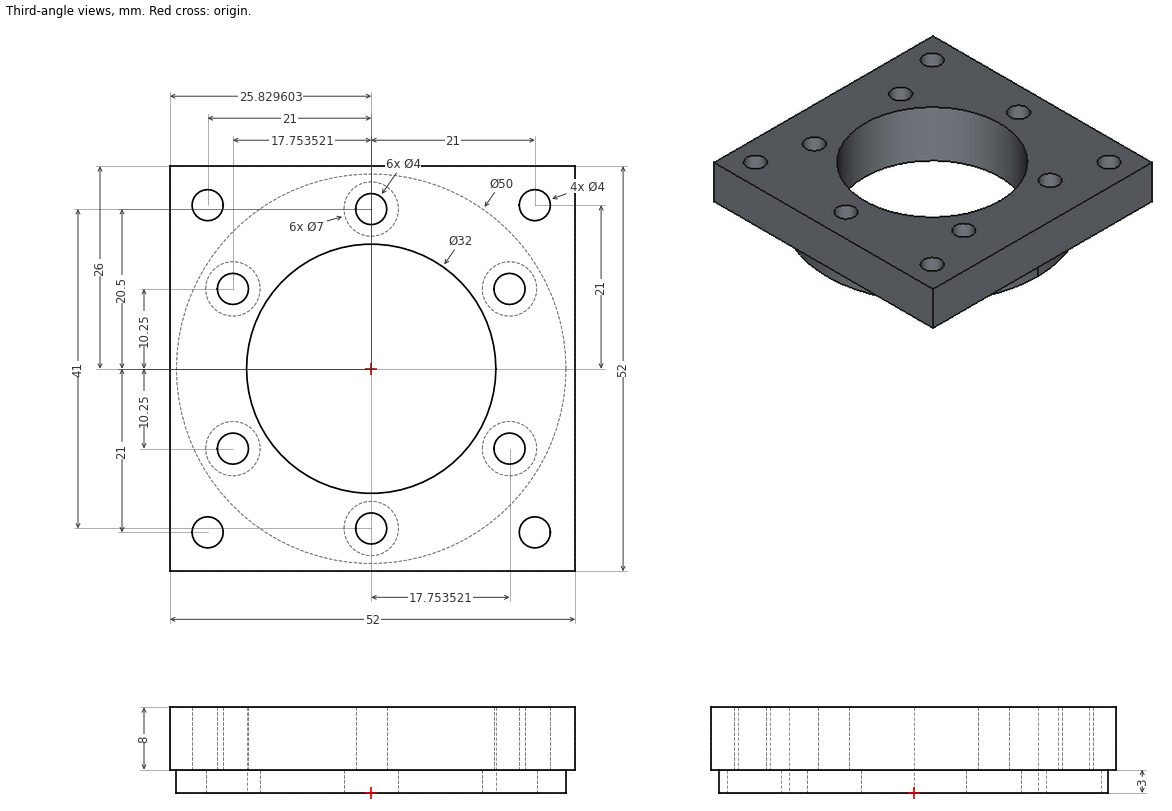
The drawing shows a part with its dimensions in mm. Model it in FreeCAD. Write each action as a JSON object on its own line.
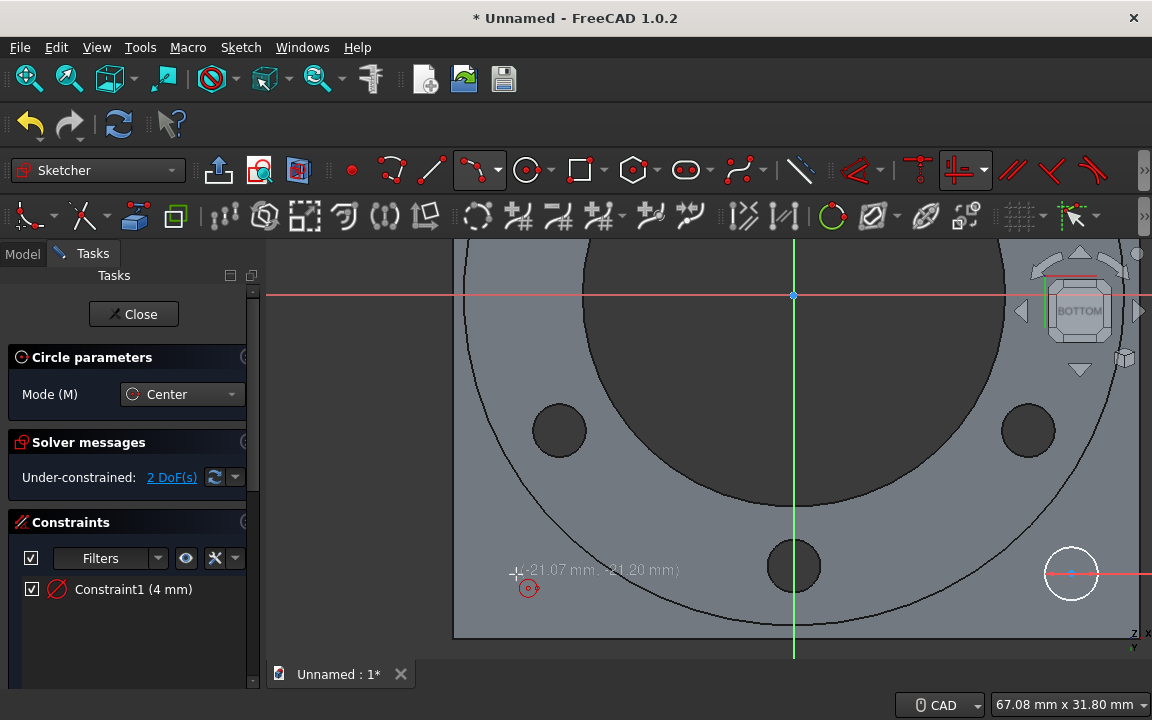
{"action": "left_click", "coordinate": [517, 573]}
{"action": "mouse_move", "coordinate": [535, 554]}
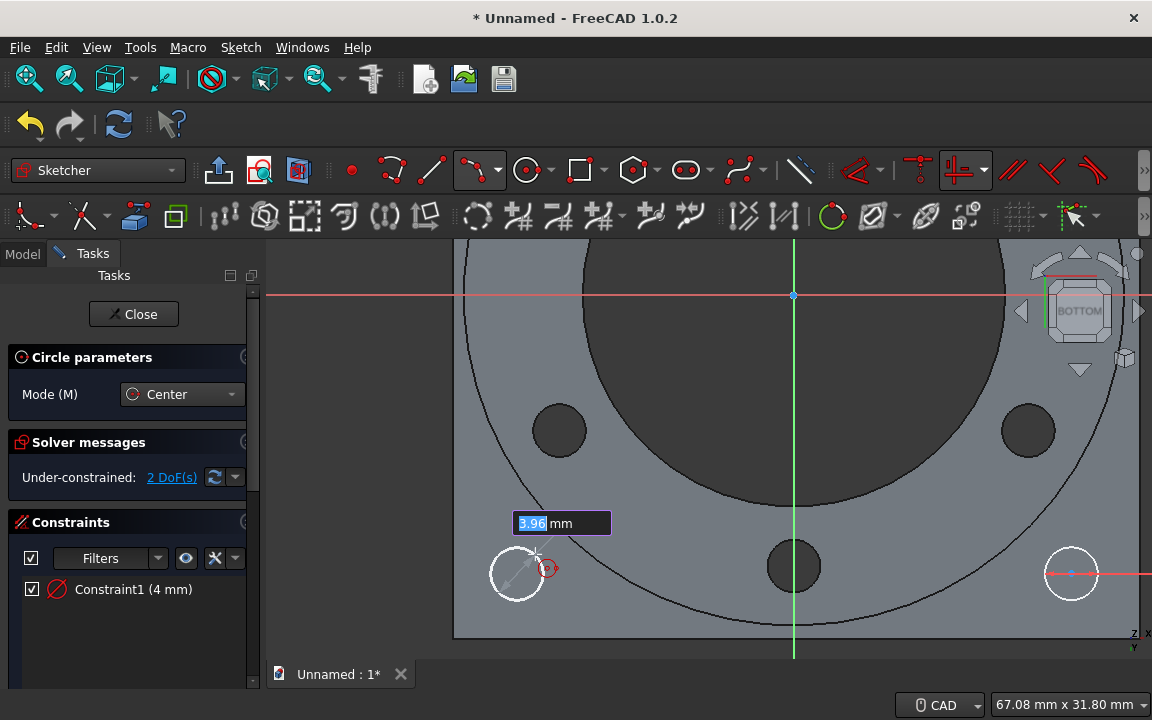
{"action": "type", "text": "4"}
{"action": "key", "text": "Return"}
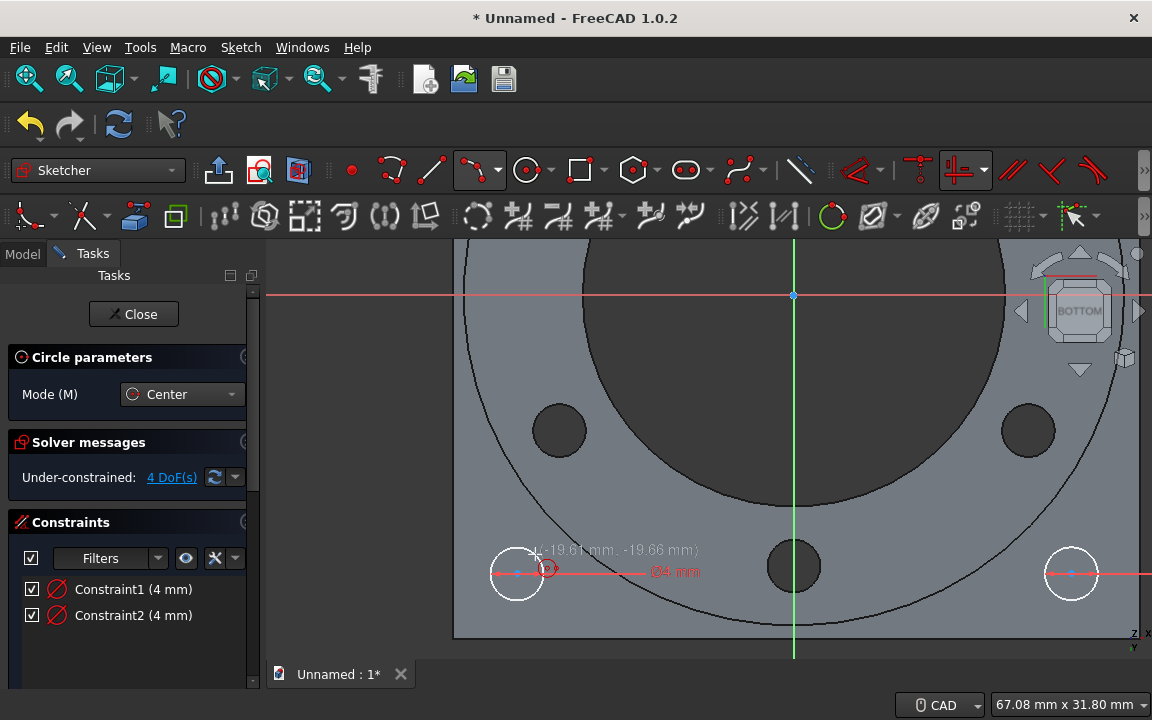
{"action": "scroll", "coordinate": [515, 574], "scroll_direction": "down", "scroll_amount": 4}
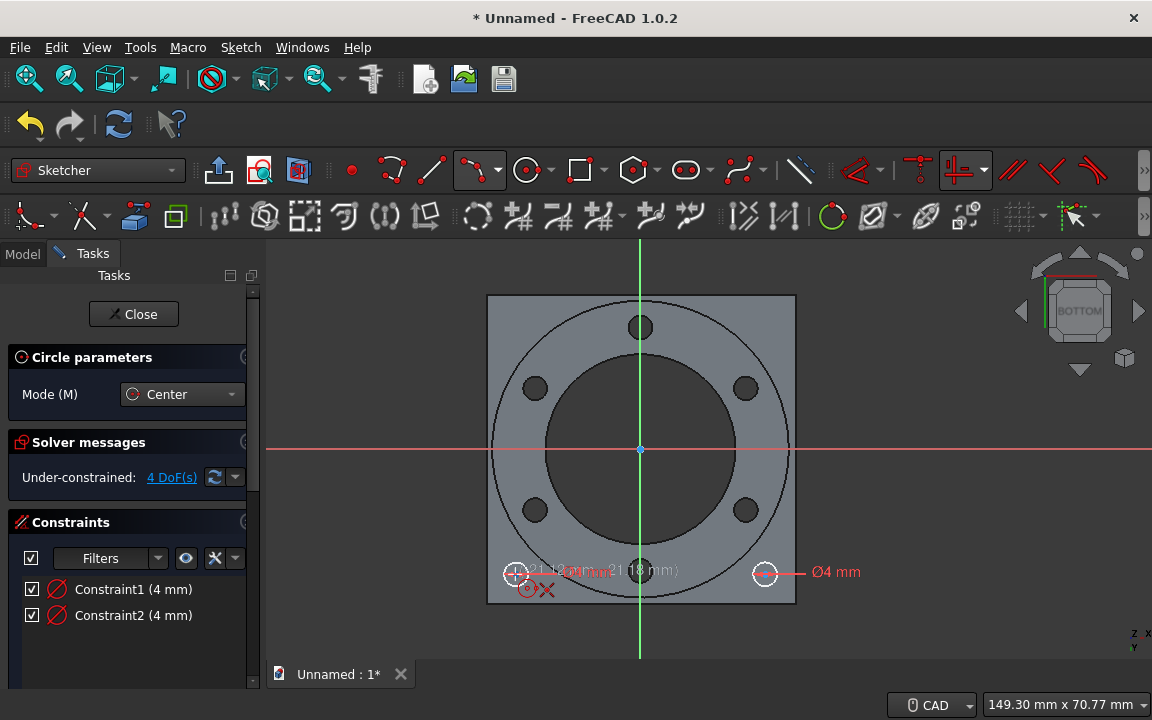
{"action": "scroll", "coordinate": [516, 325], "scroll_direction": "up", "scroll_amount": 4}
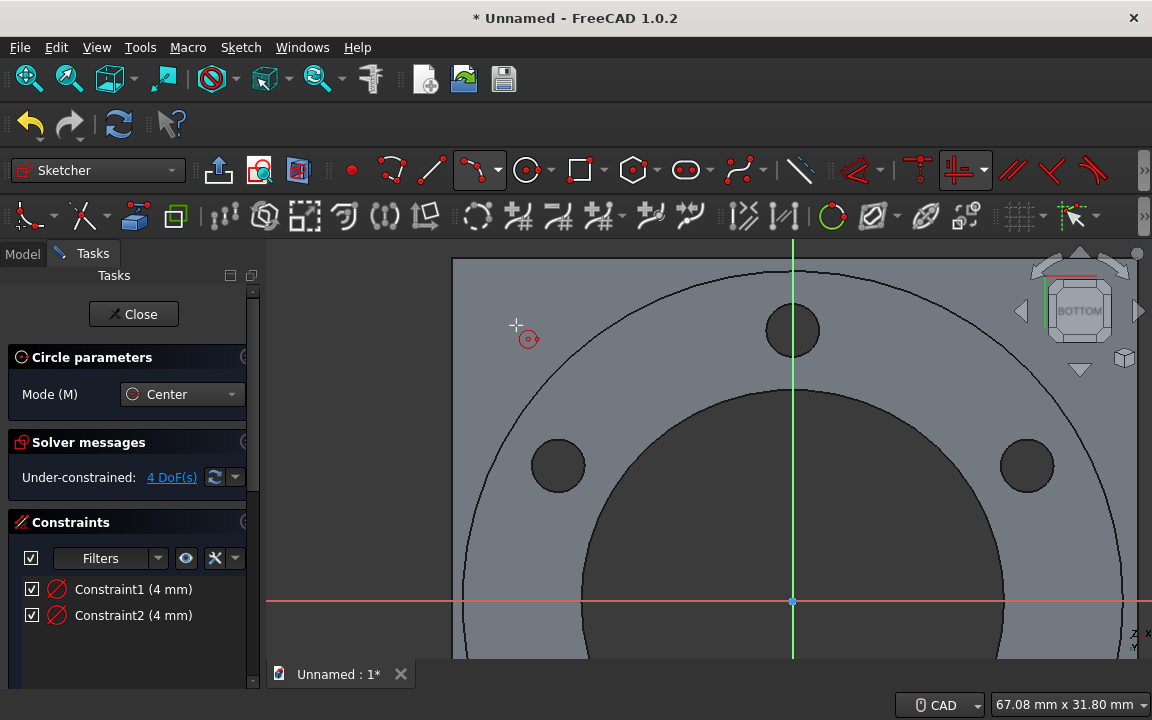
{"action": "left_click", "coordinate": [515, 324]}
{"action": "mouse_move", "coordinate": [534, 305]}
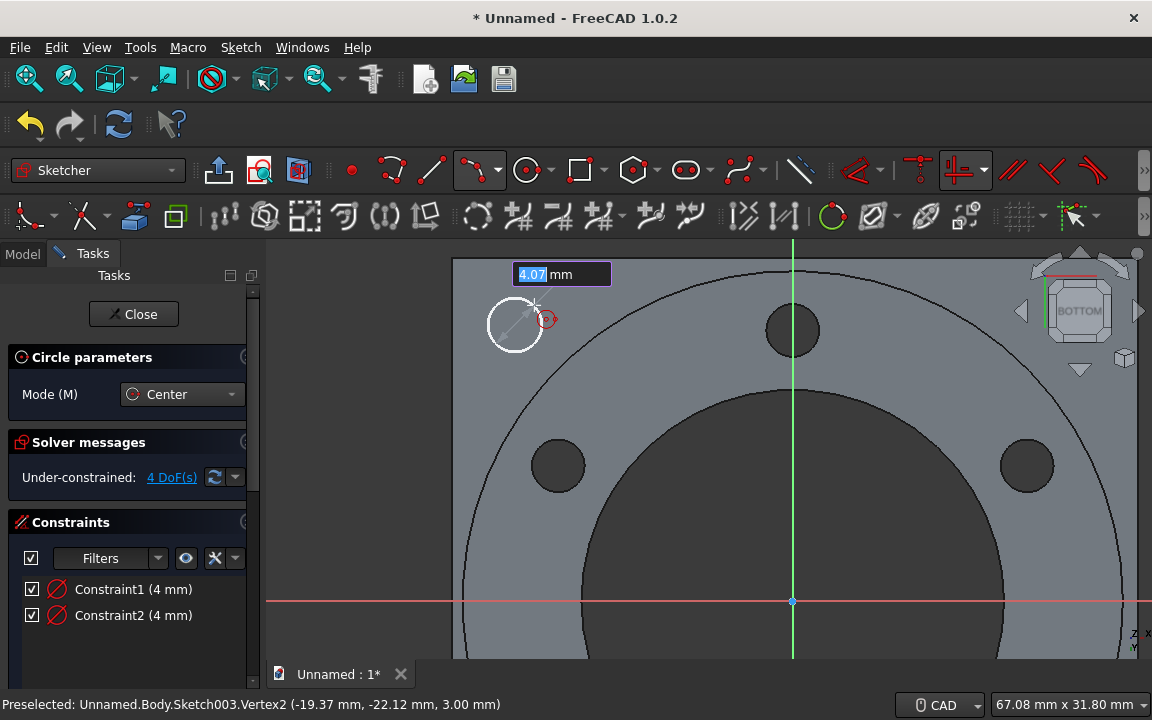
{"action": "type", "text": "4"}
{"action": "key", "text": "Return"}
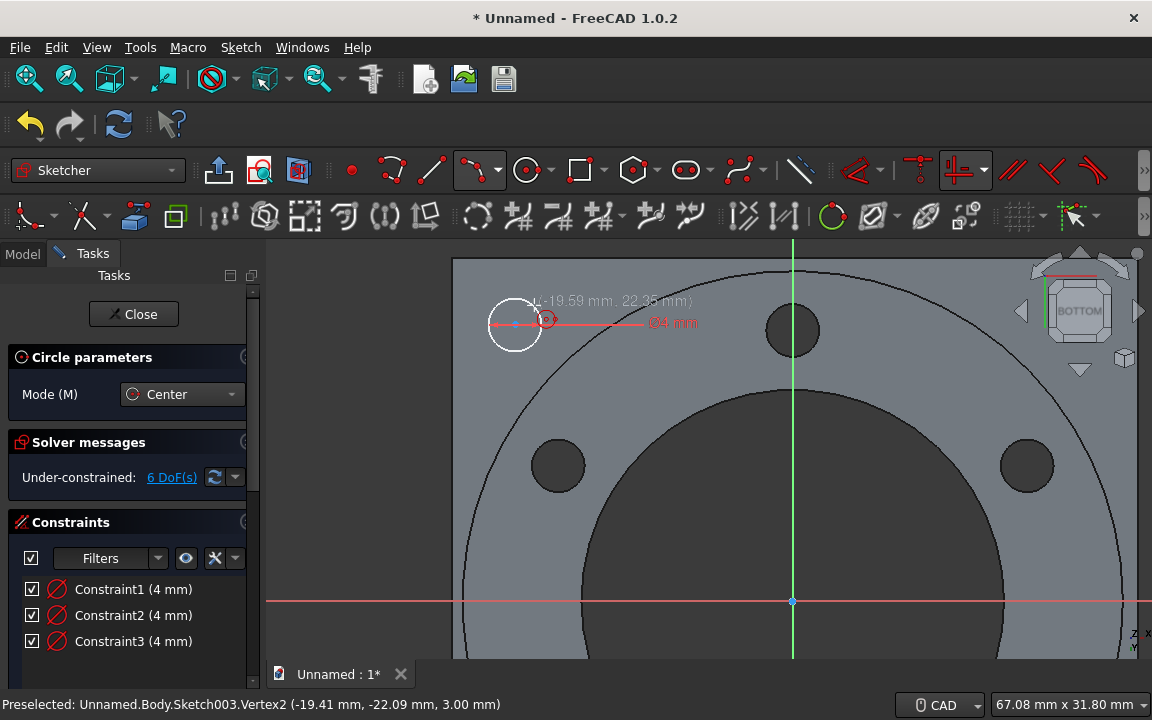
{"action": "scroll", "coordinate": [516, 325], "scroll_direction": "down", "scroll_amount": 4}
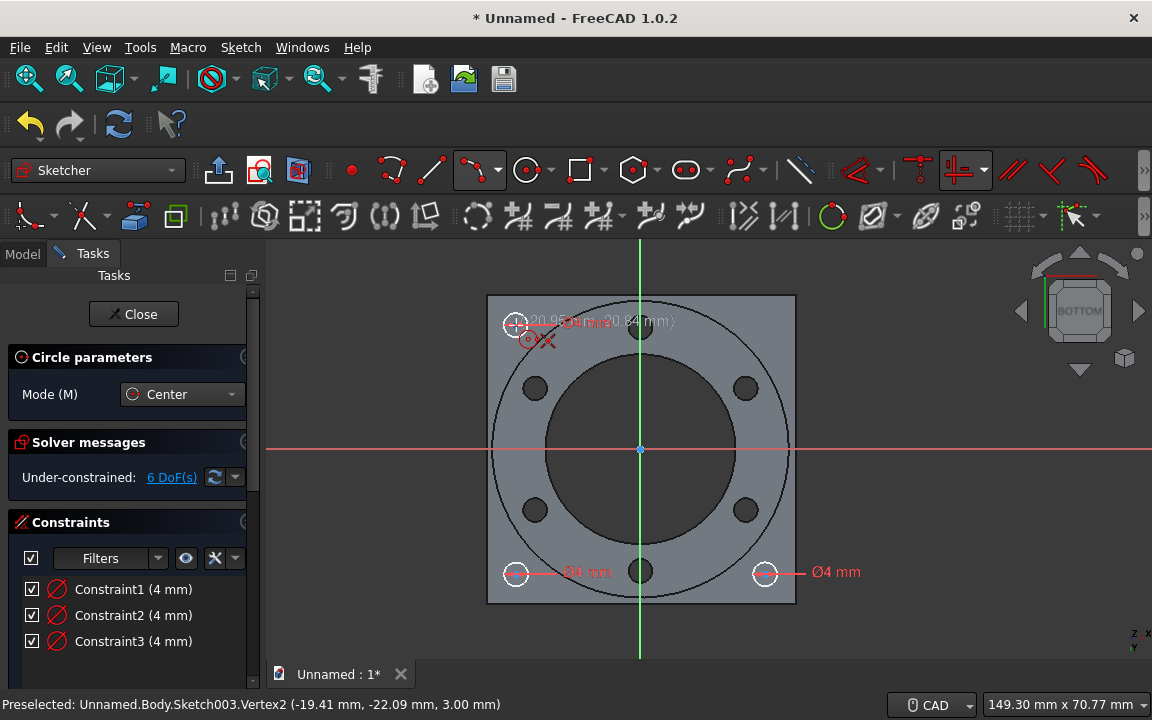
{"action": "scroll", "coordinate": [765, 325], "scroll_direction": "up", "scroll_amount": 4}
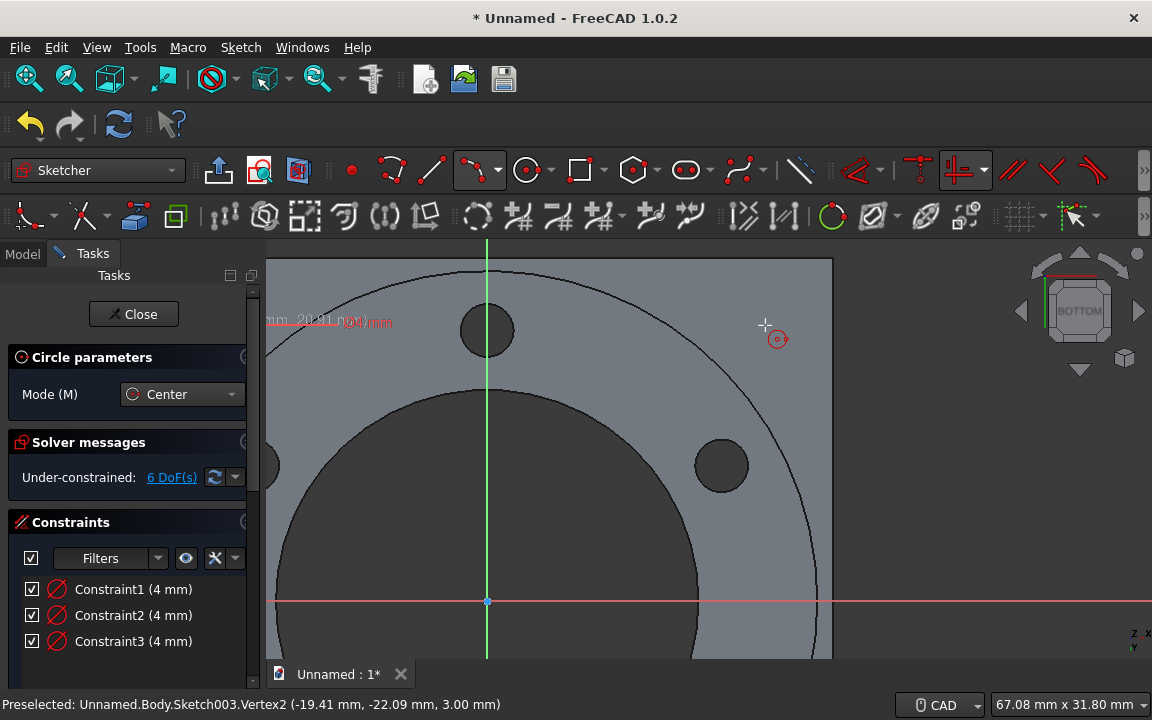
{"action": "left_click", "coordinate": [765, 324]}
{"action": "mouse_move", "coordinate": [783, 305]}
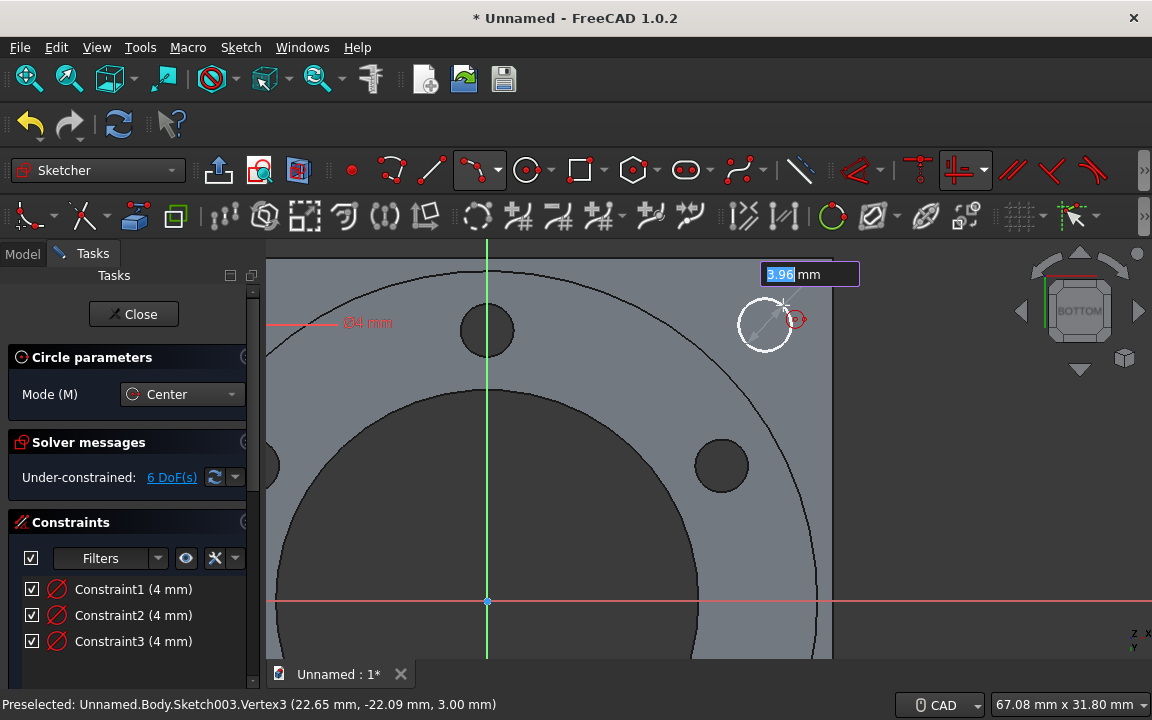
{"action": "type", "text": "4"}
{"action": "key", "text": "Return"}
{"action": "key", "text": "Escape"}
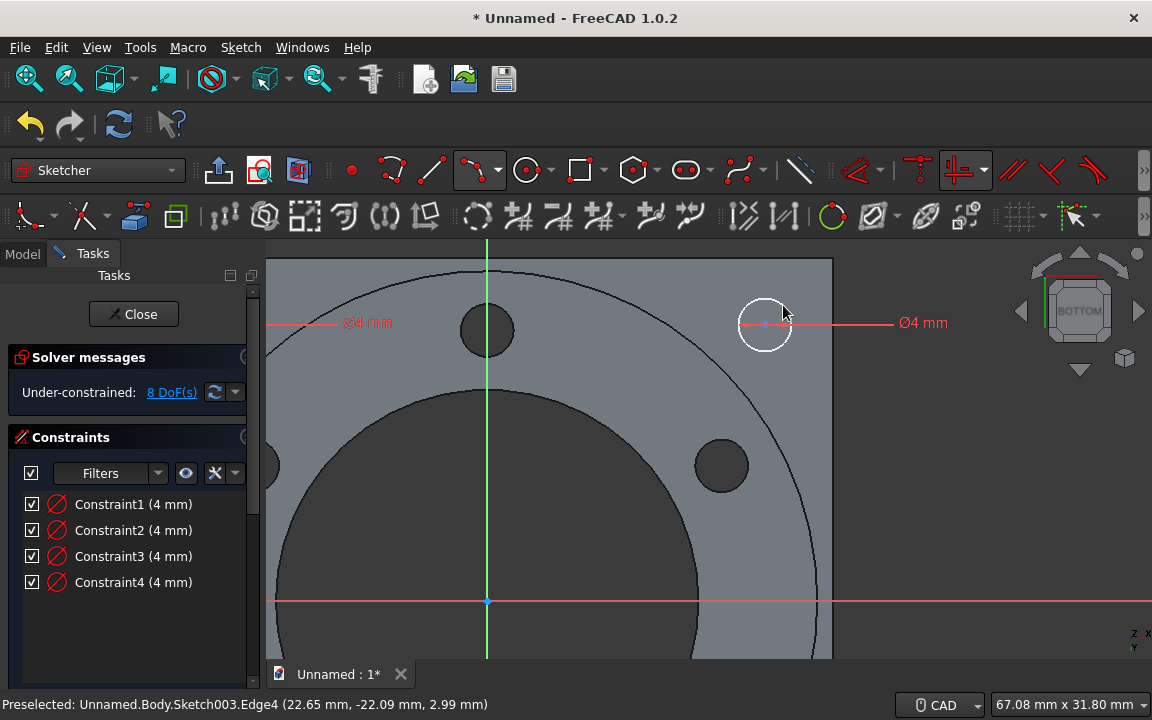
{"action": "scroll", "coordinate": [766, 325], "scroll_direction": "down", "scroll_amount": 4}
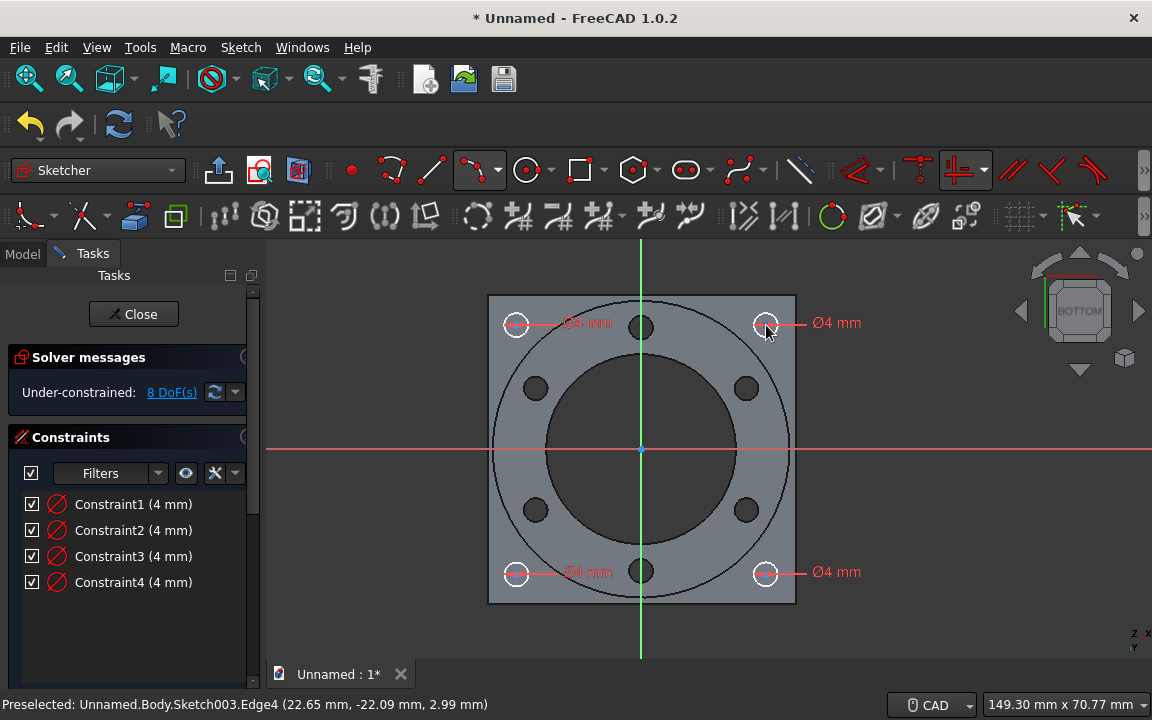
{"action": "left_click", "coordinate": [766, 574]}